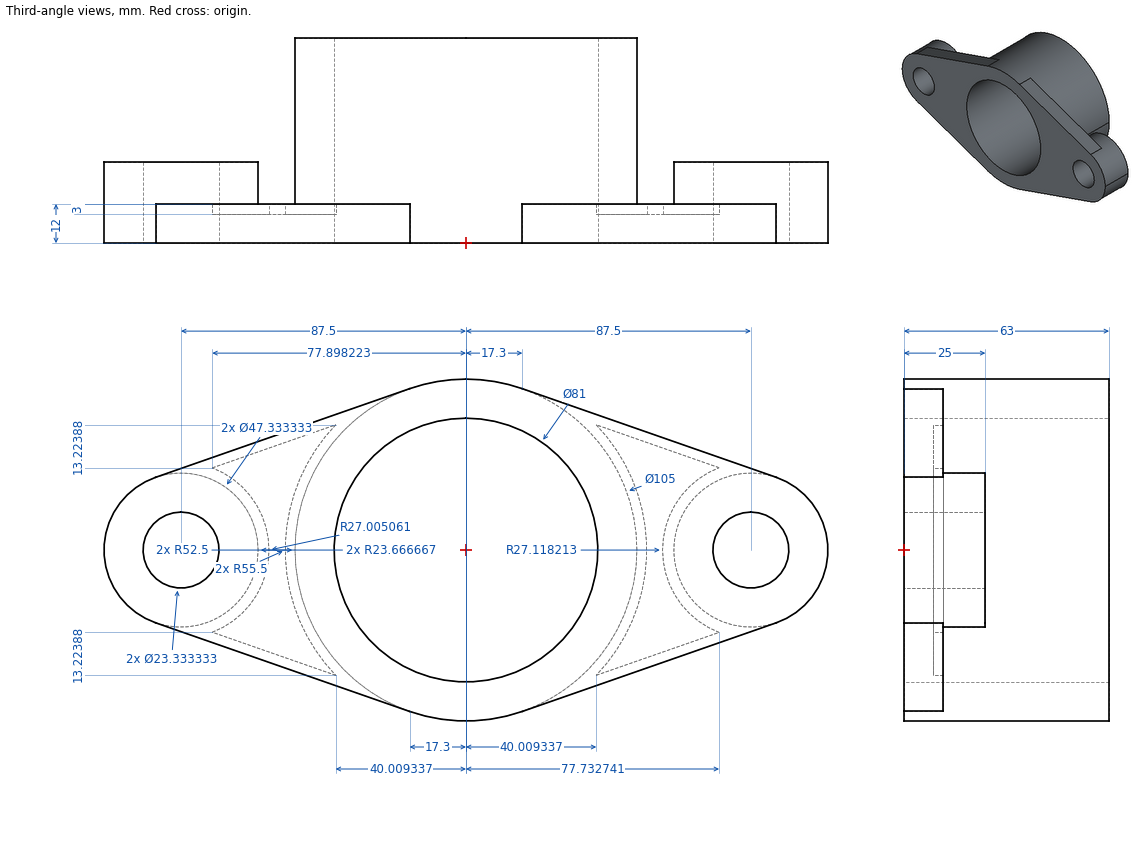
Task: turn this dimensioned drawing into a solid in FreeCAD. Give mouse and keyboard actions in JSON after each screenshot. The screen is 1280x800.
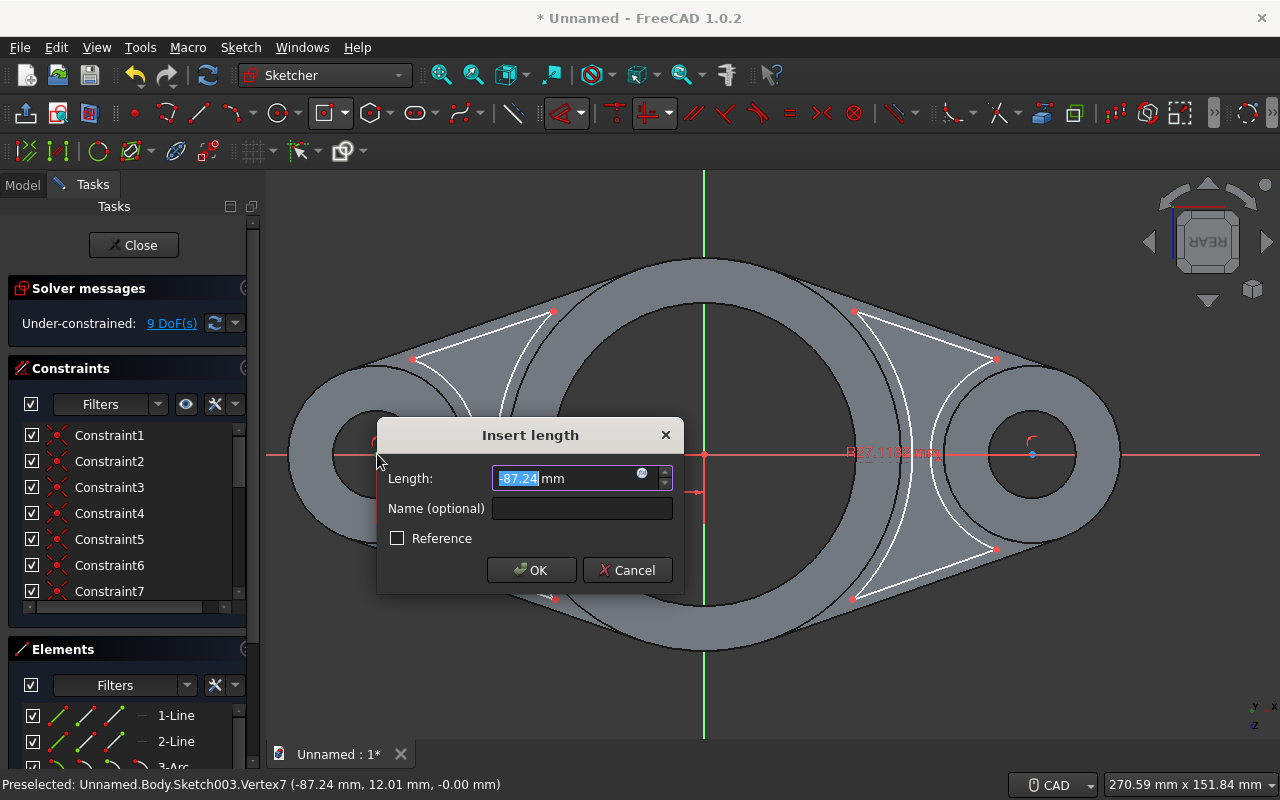
{"action": "type", "text": "-87.5"}
{"action": "key", "text": "Return"}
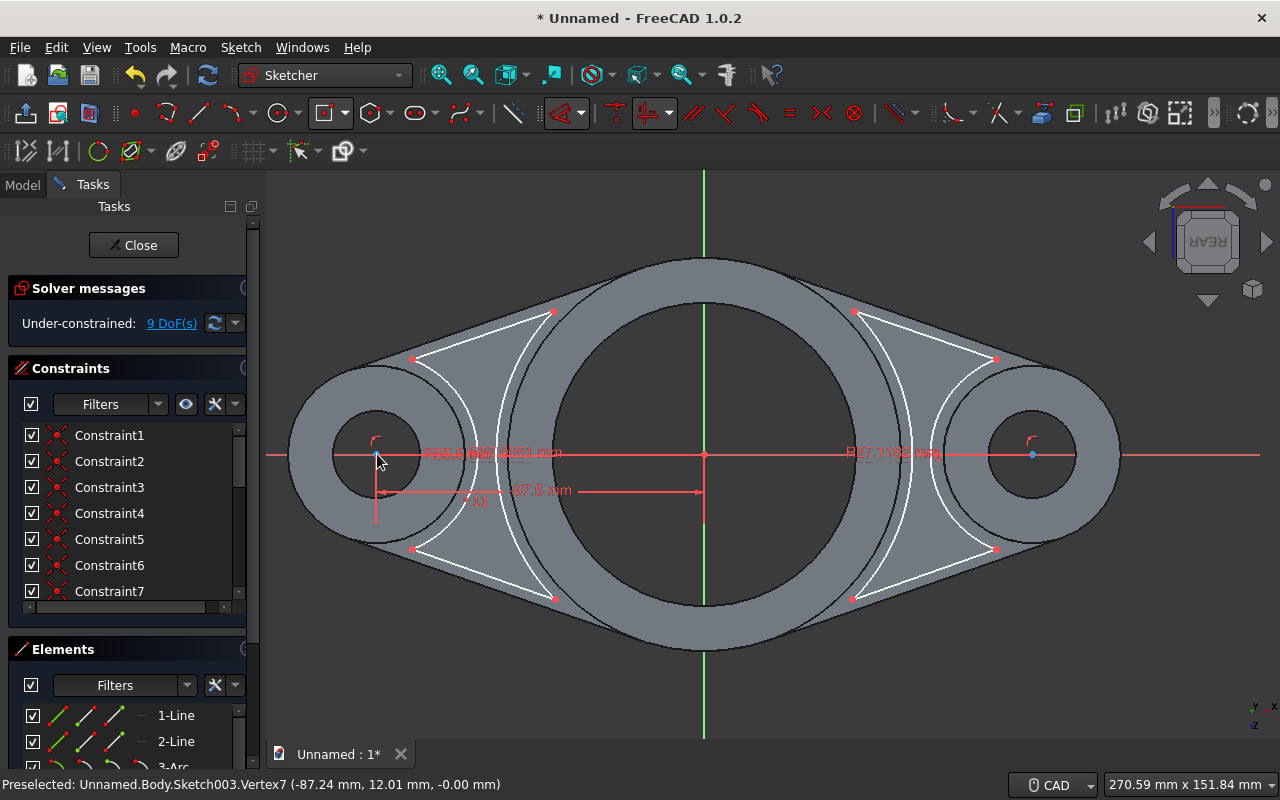
{"action": "left_click", "coordinate": [1032, 454]}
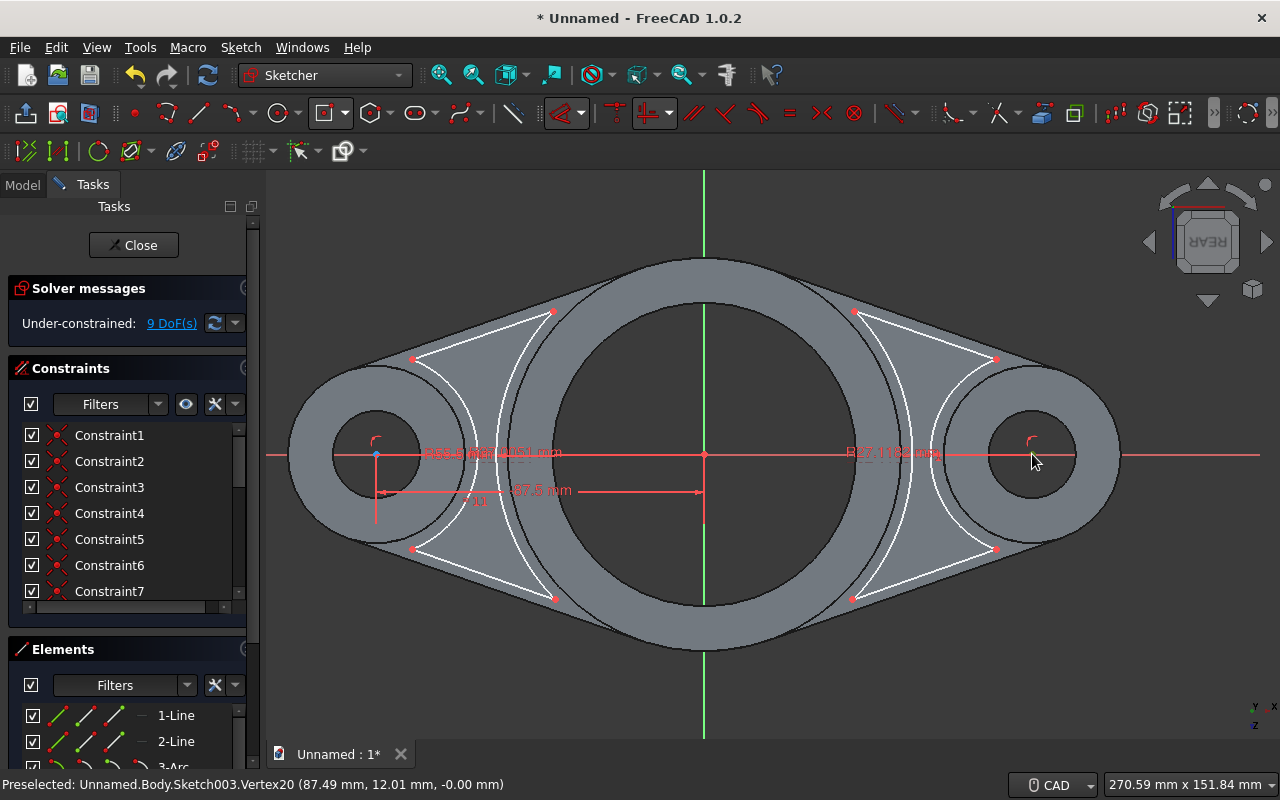
{"action": "key", "text": "l"}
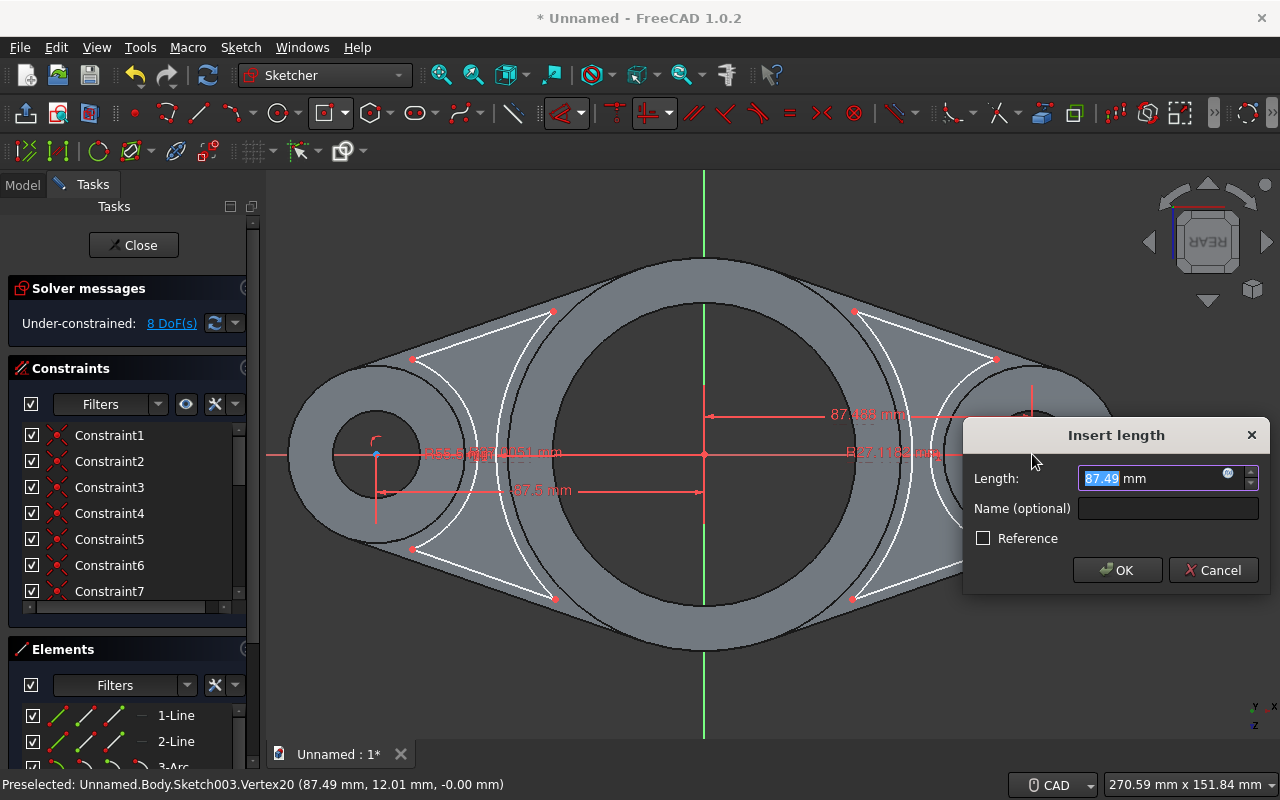
{"action": "type", "text": "87.5"}
{"action": "key", "text": "Return"}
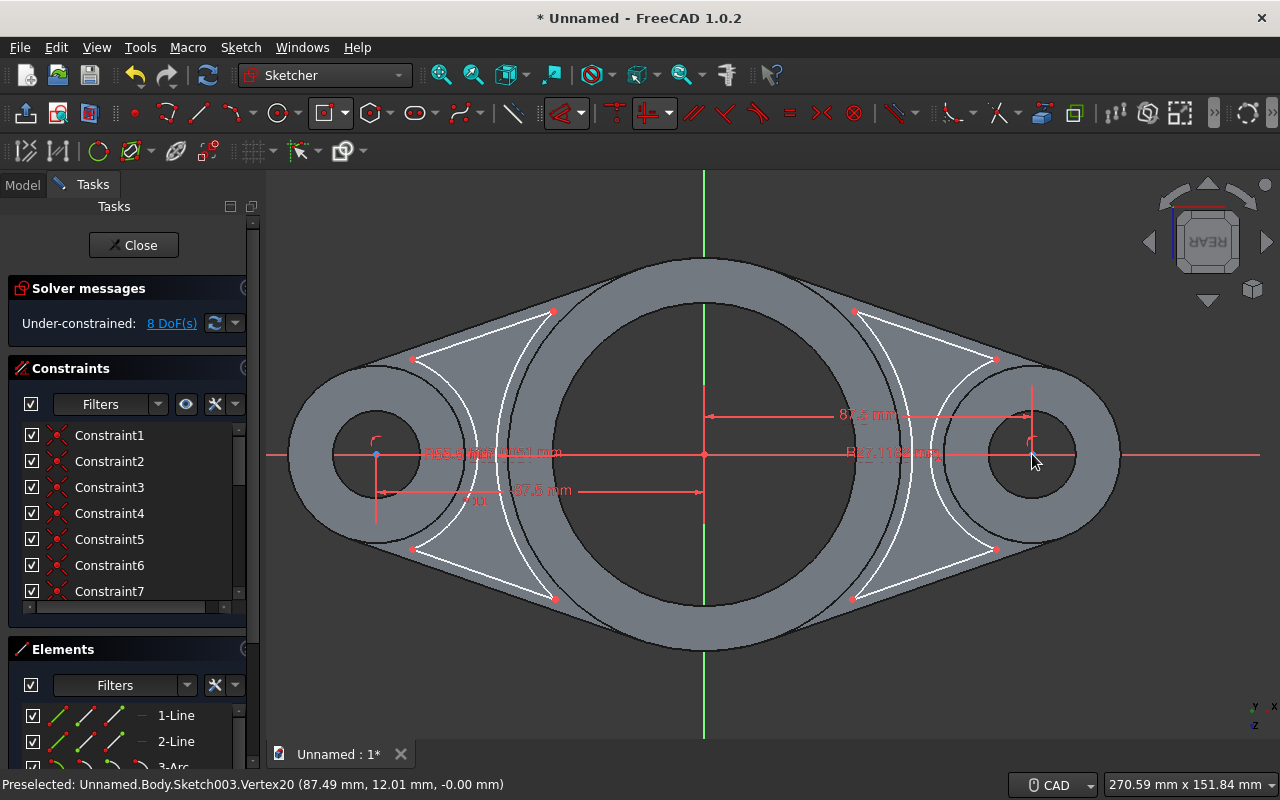
{"action": "left_click", "coordinate": [511, 326]}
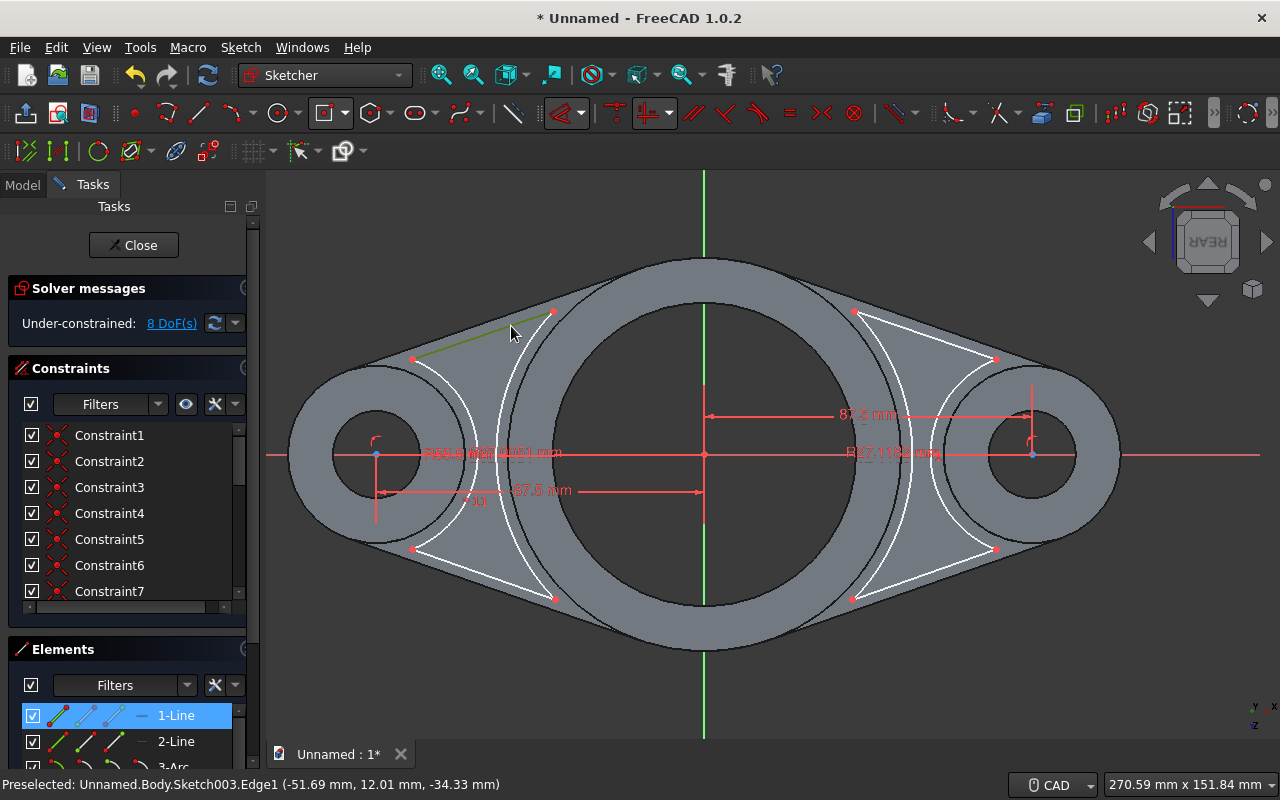
{"action": "key", "text": "i"}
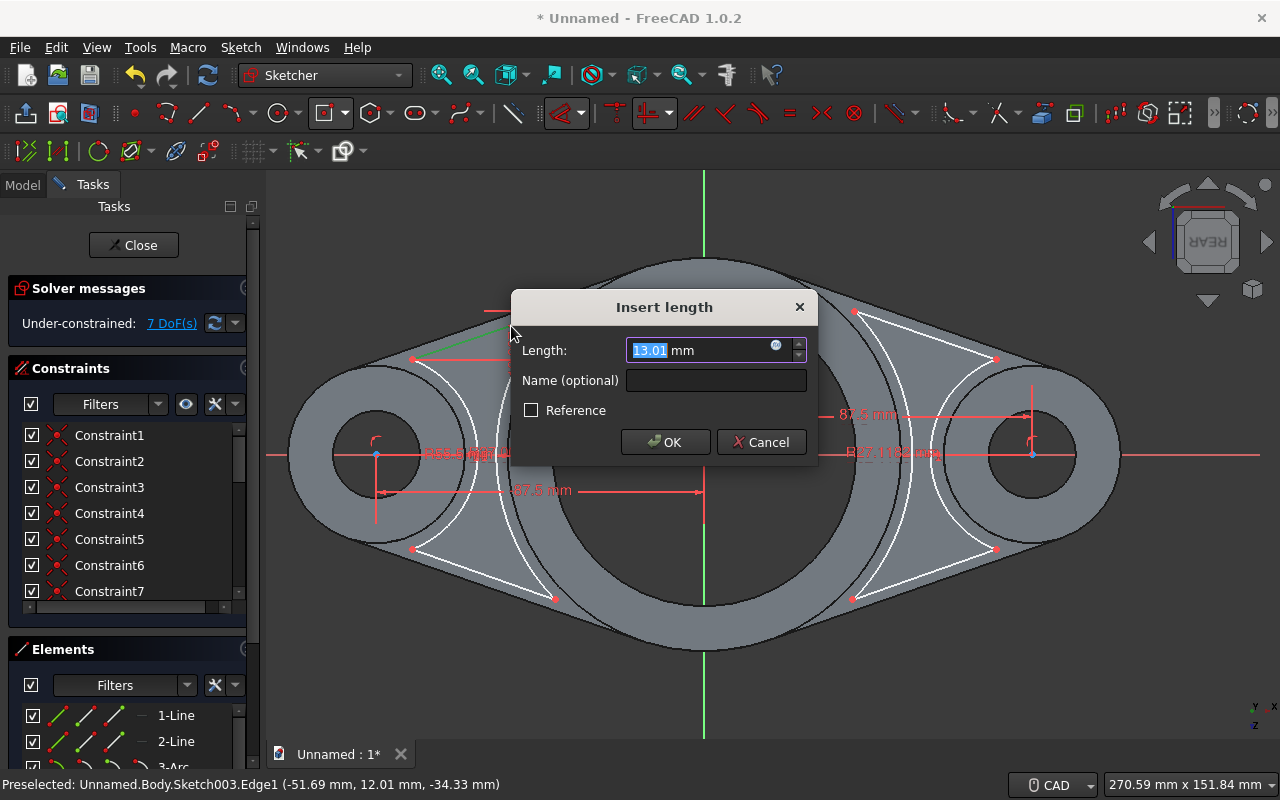
{"action": "type", "text": "13.22388"}
{"action": "key", "text": "Return"}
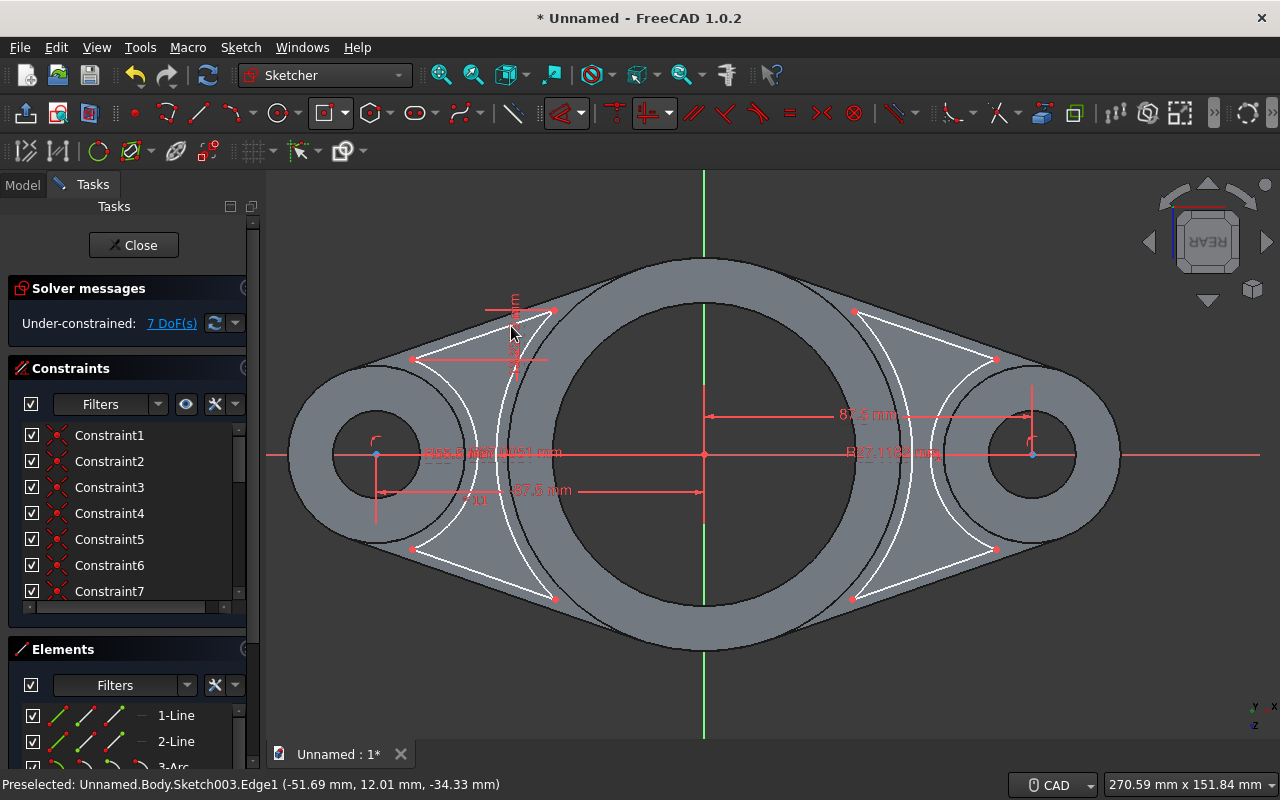
{"action": "left_click", "coordinate": [455, 564]}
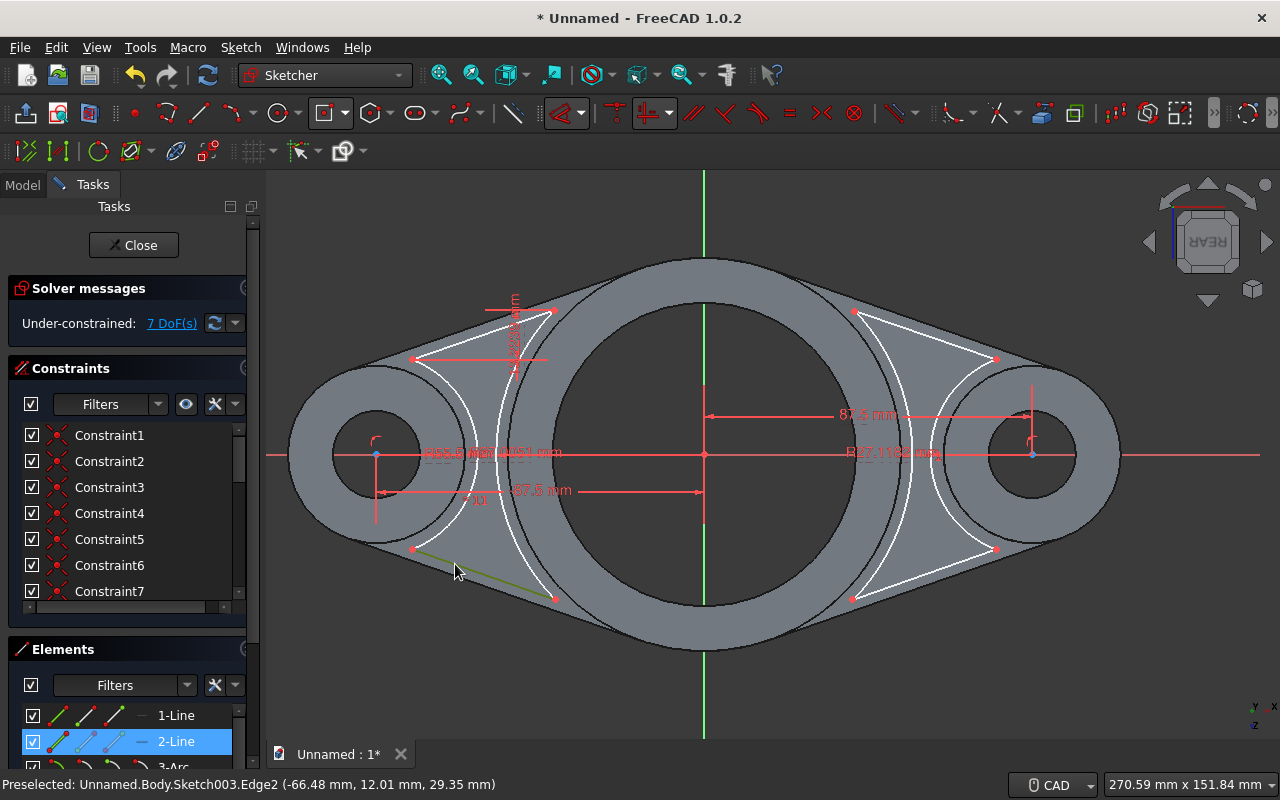
{"action": "key", "text": "i"}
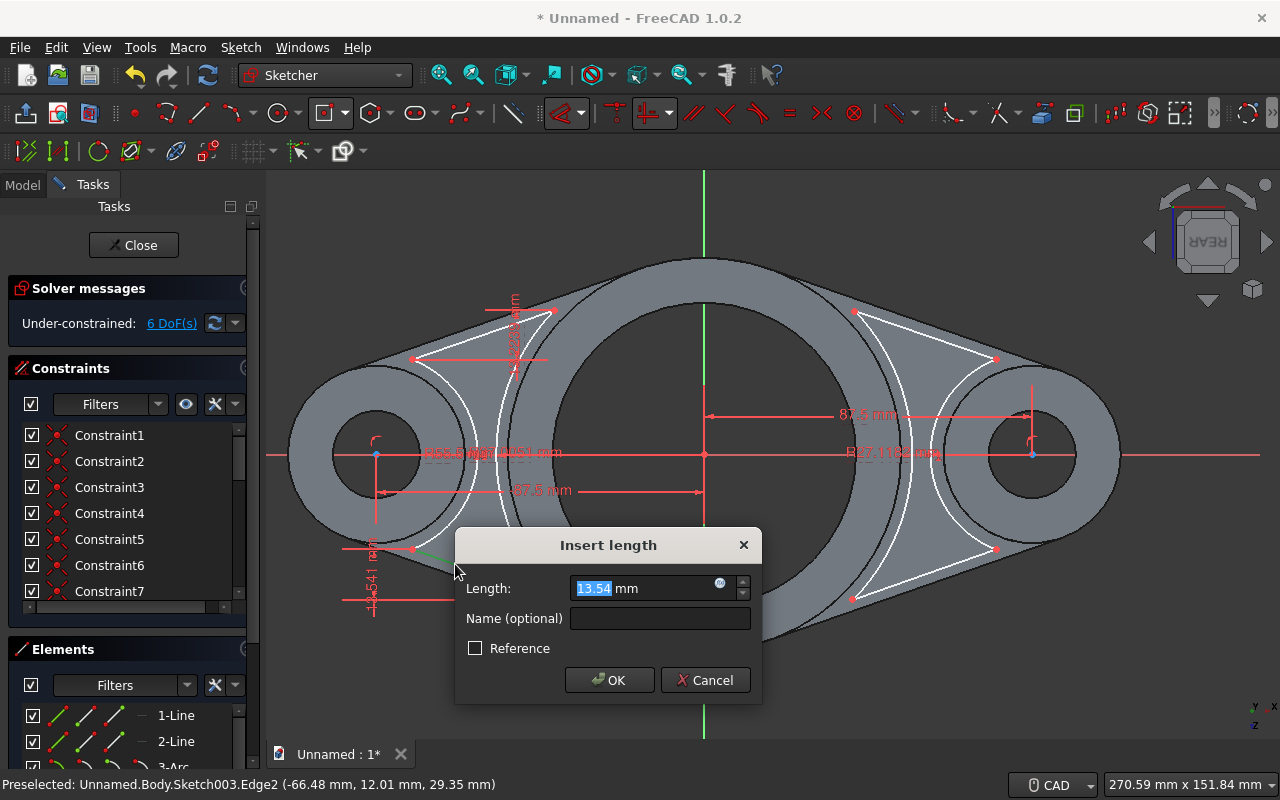
{"action": "type", "text": "13.22388"}
{"action": "key", "text": "Return"}